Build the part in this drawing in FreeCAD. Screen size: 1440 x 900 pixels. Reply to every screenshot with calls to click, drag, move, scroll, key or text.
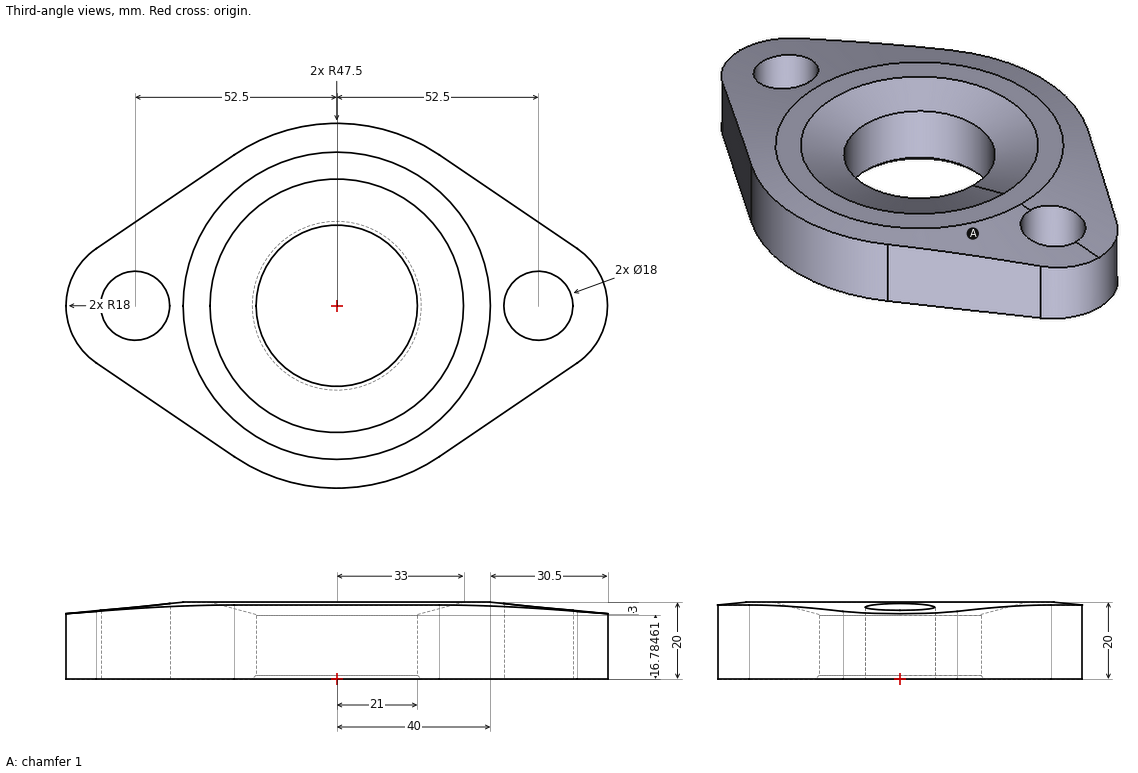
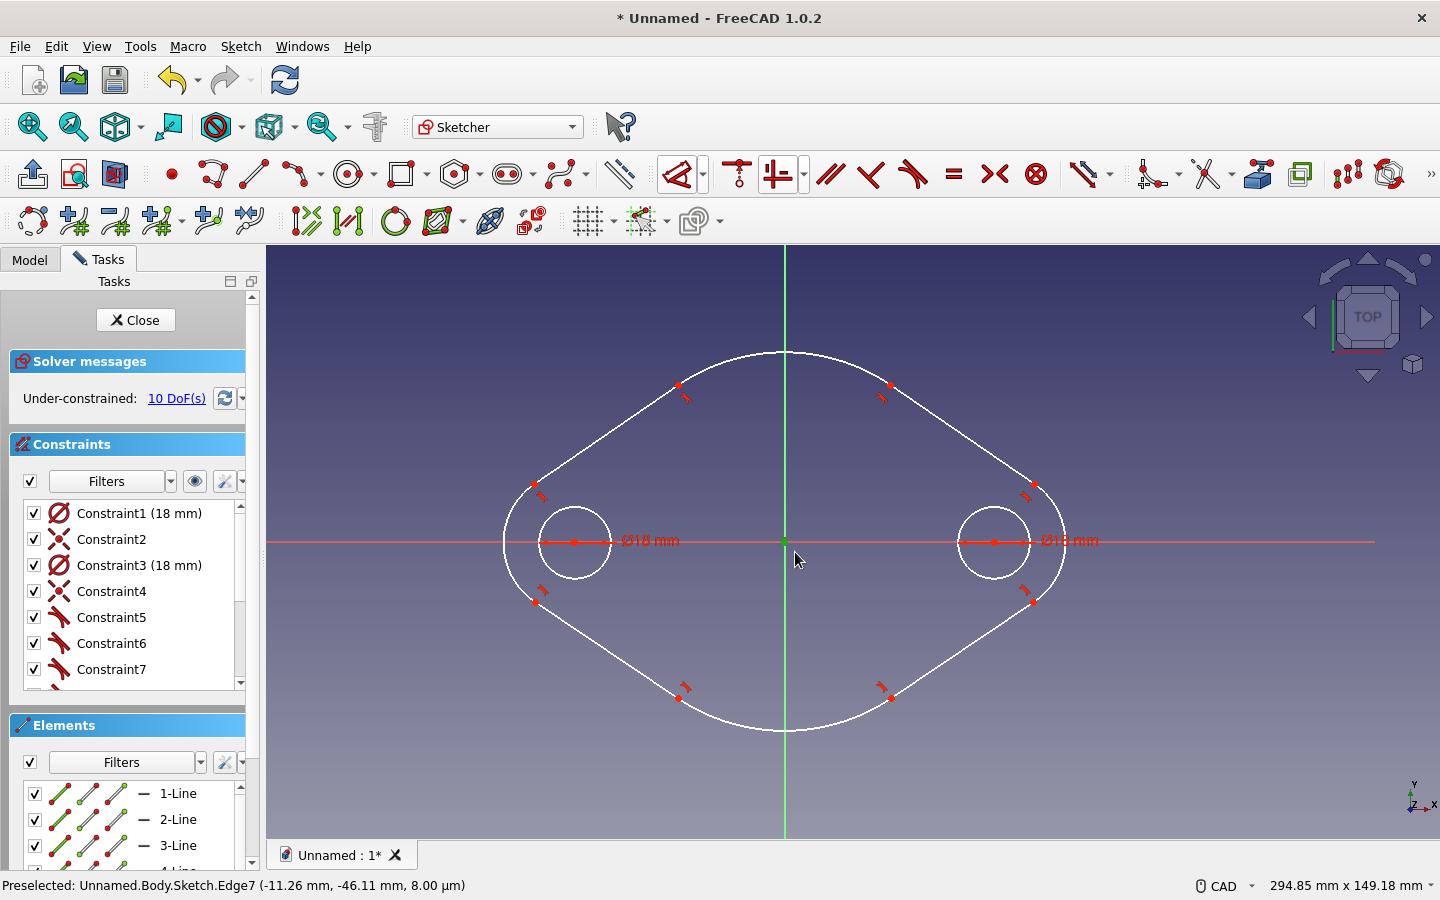
key(c)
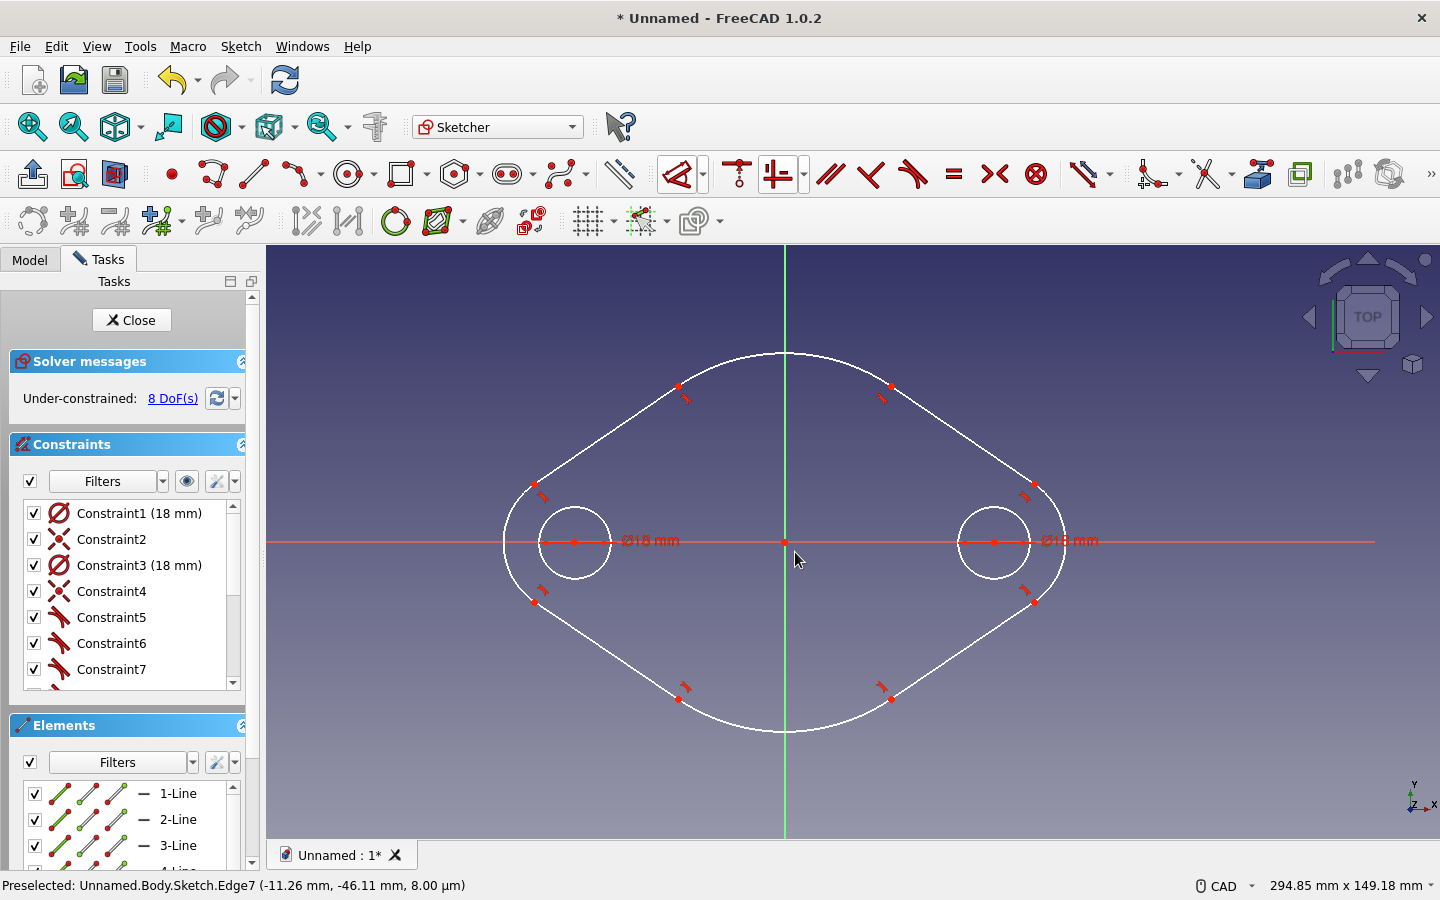
click(829, 359)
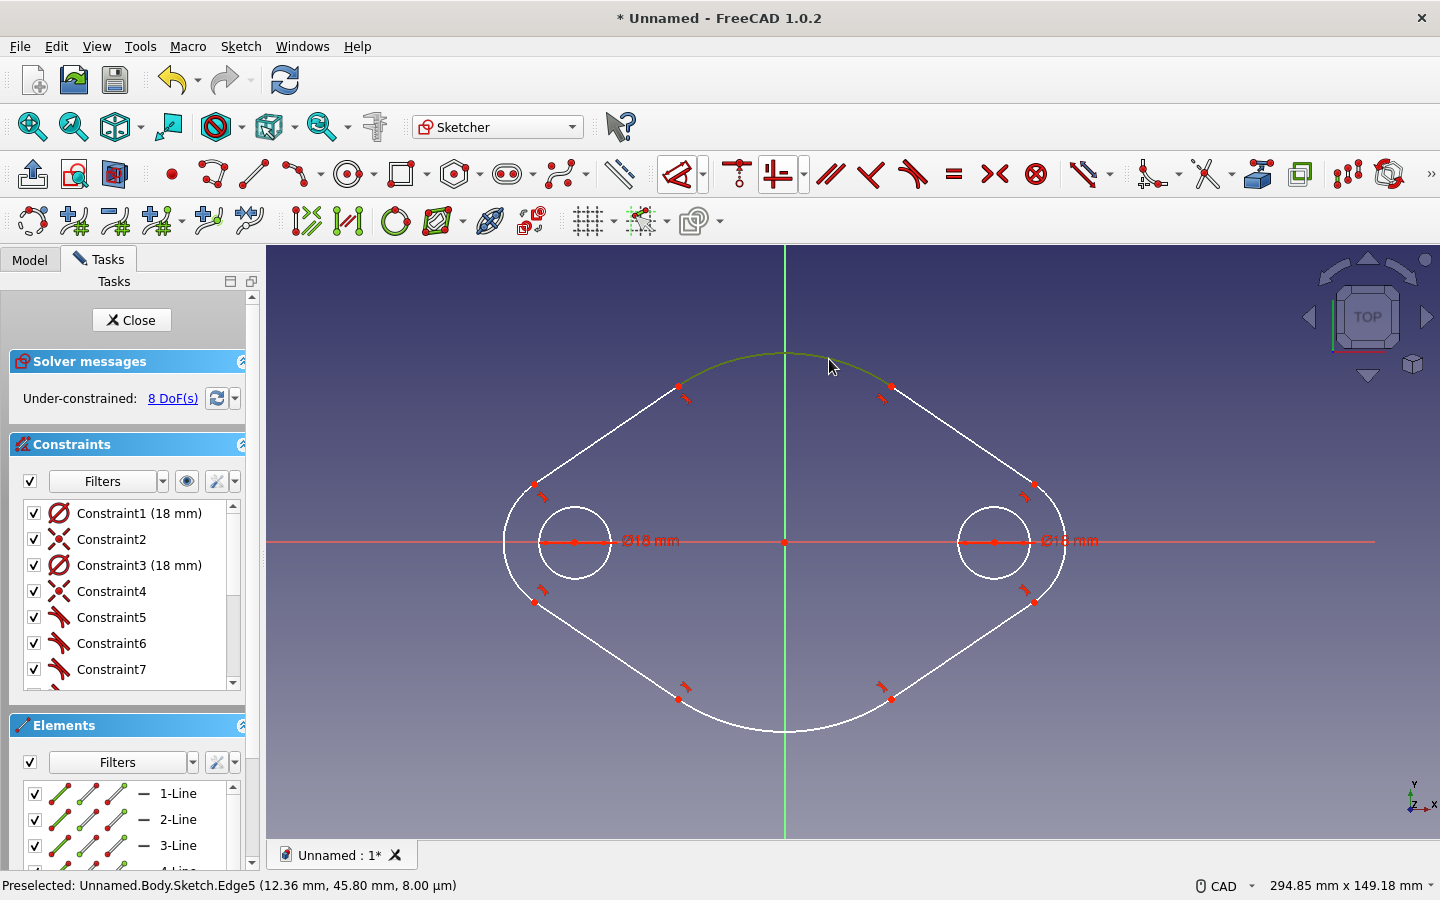
click(740, 726)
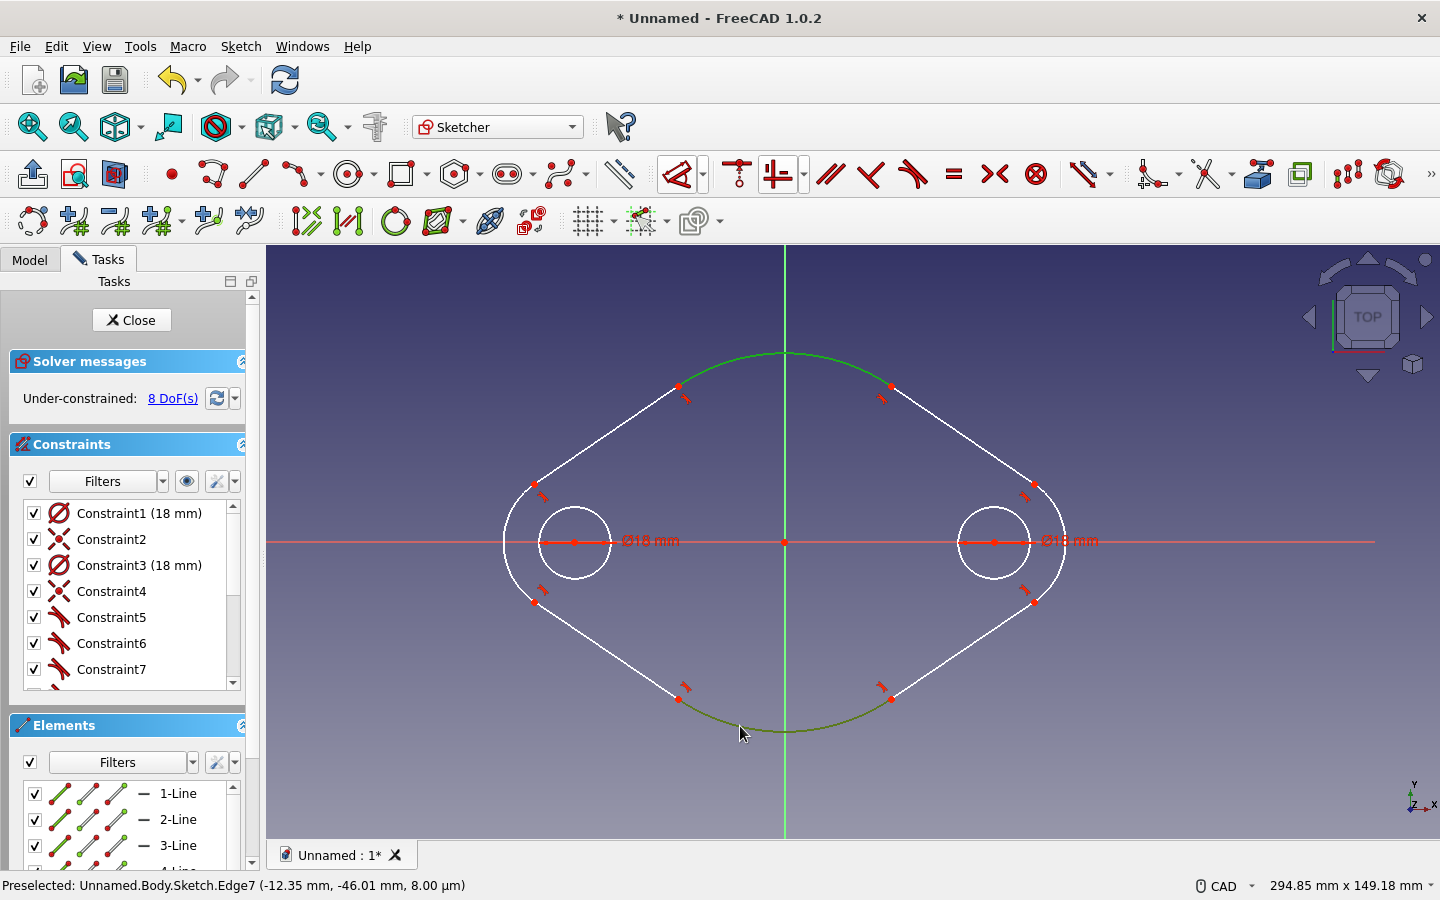
click(954, 174)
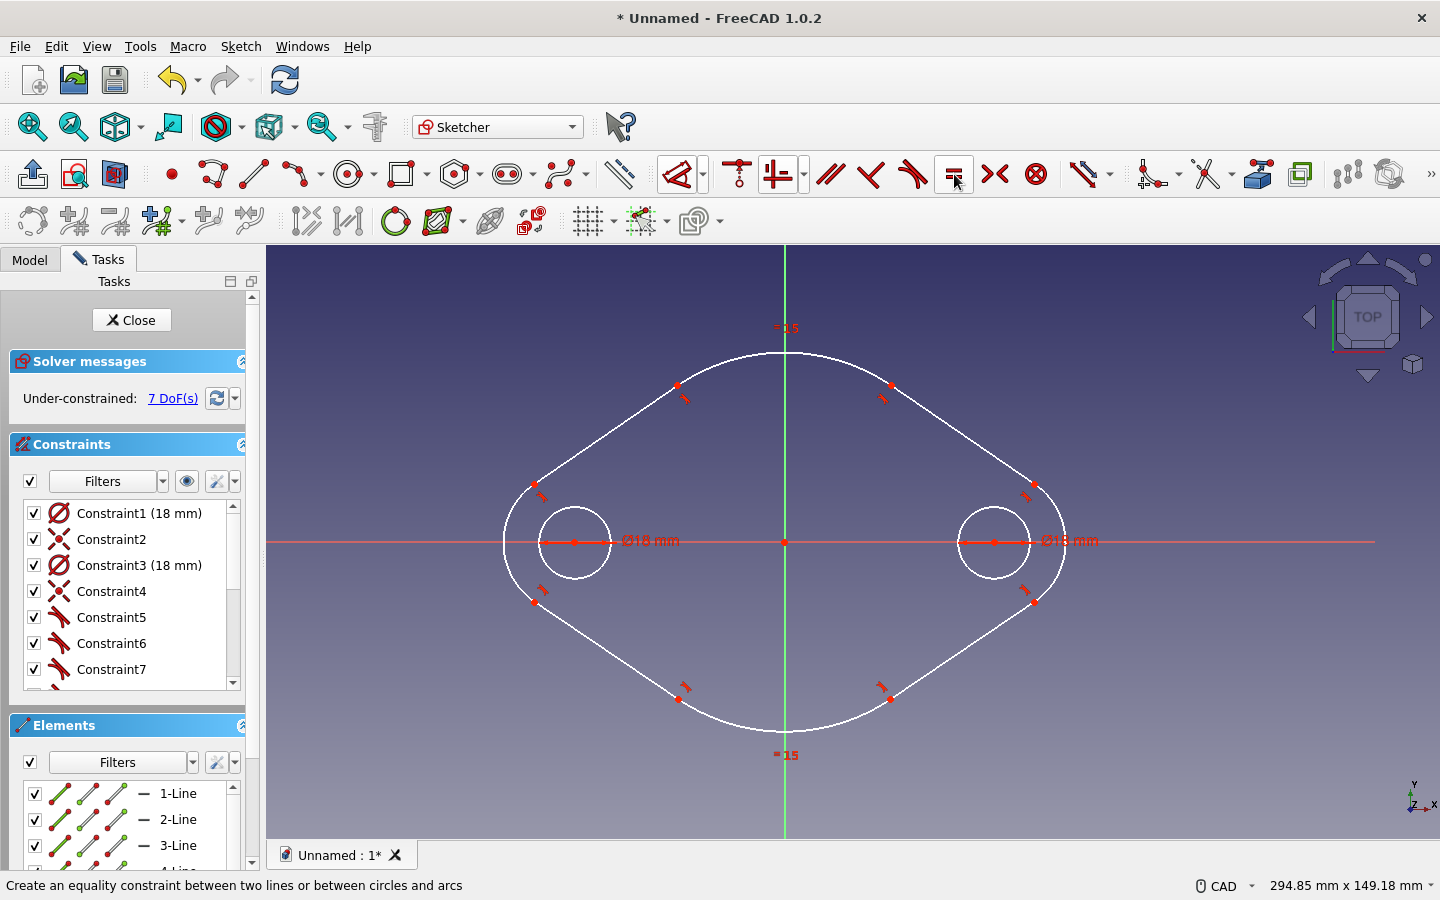
click(509, 516)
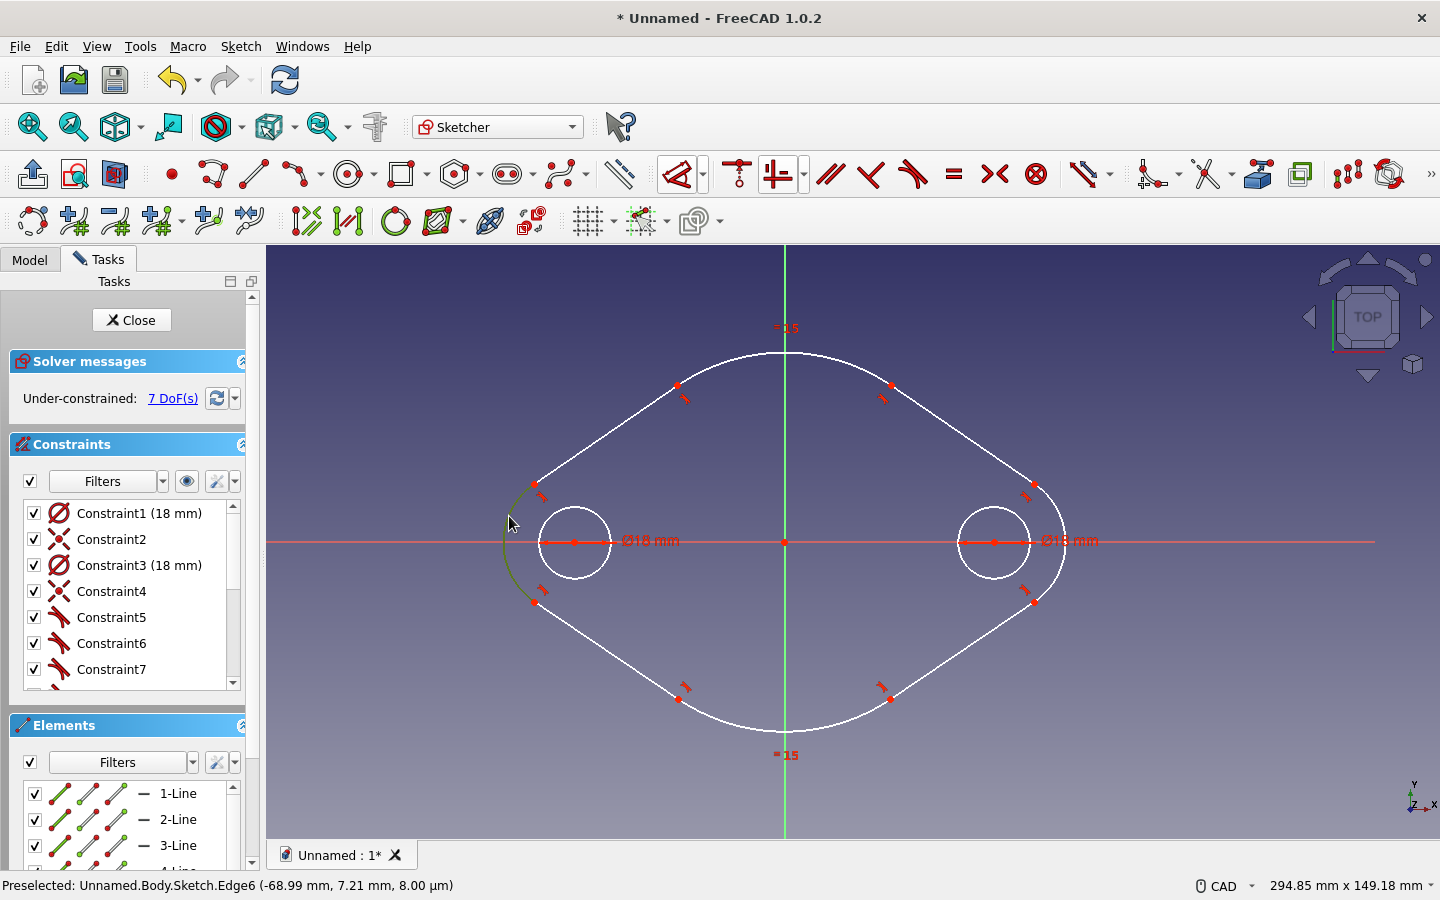
click(1060, 570)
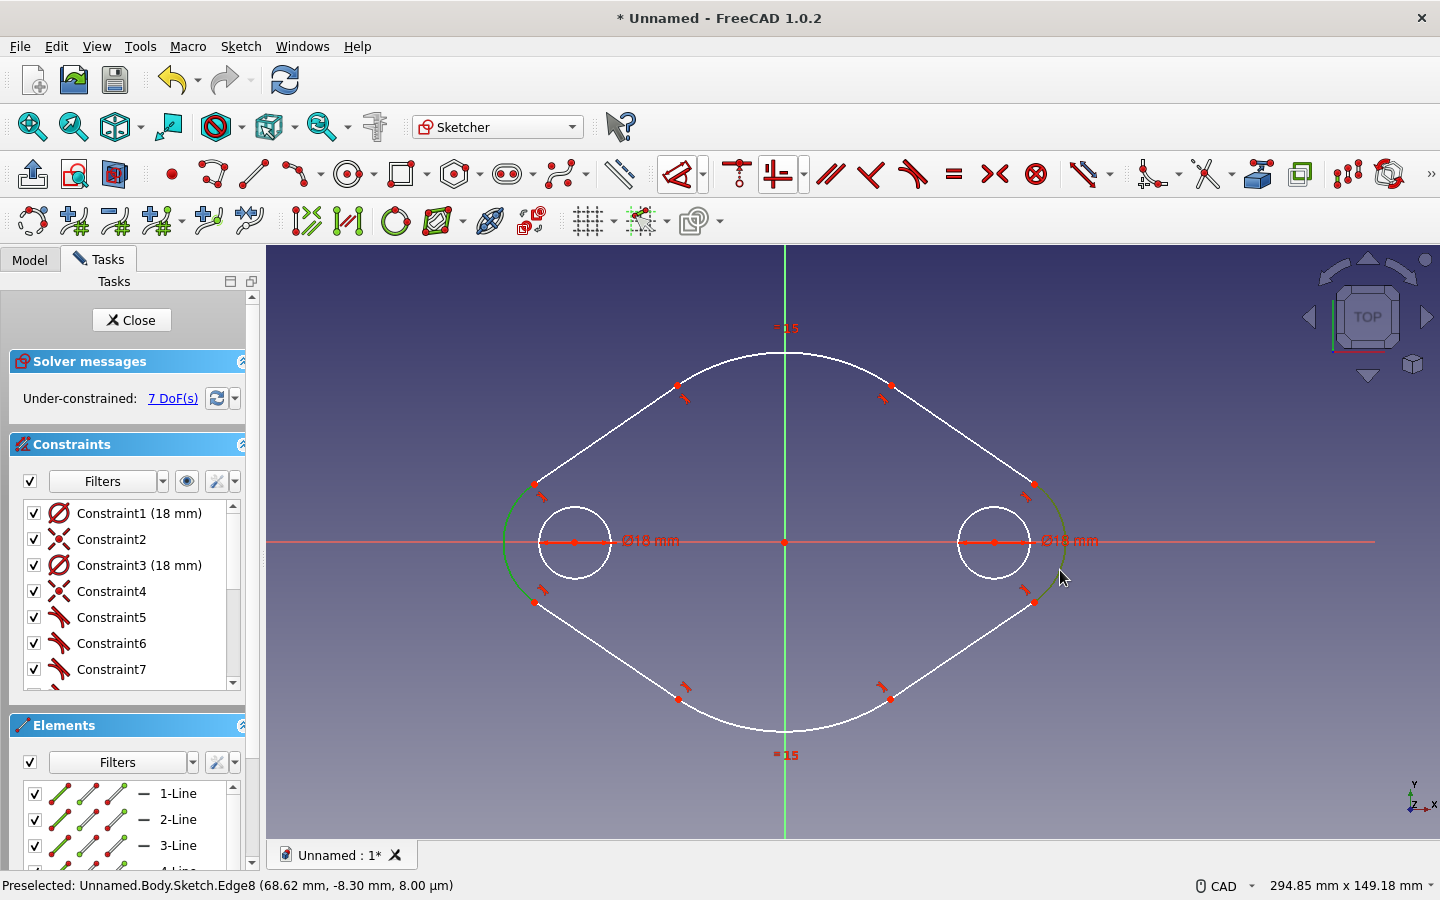
key(e)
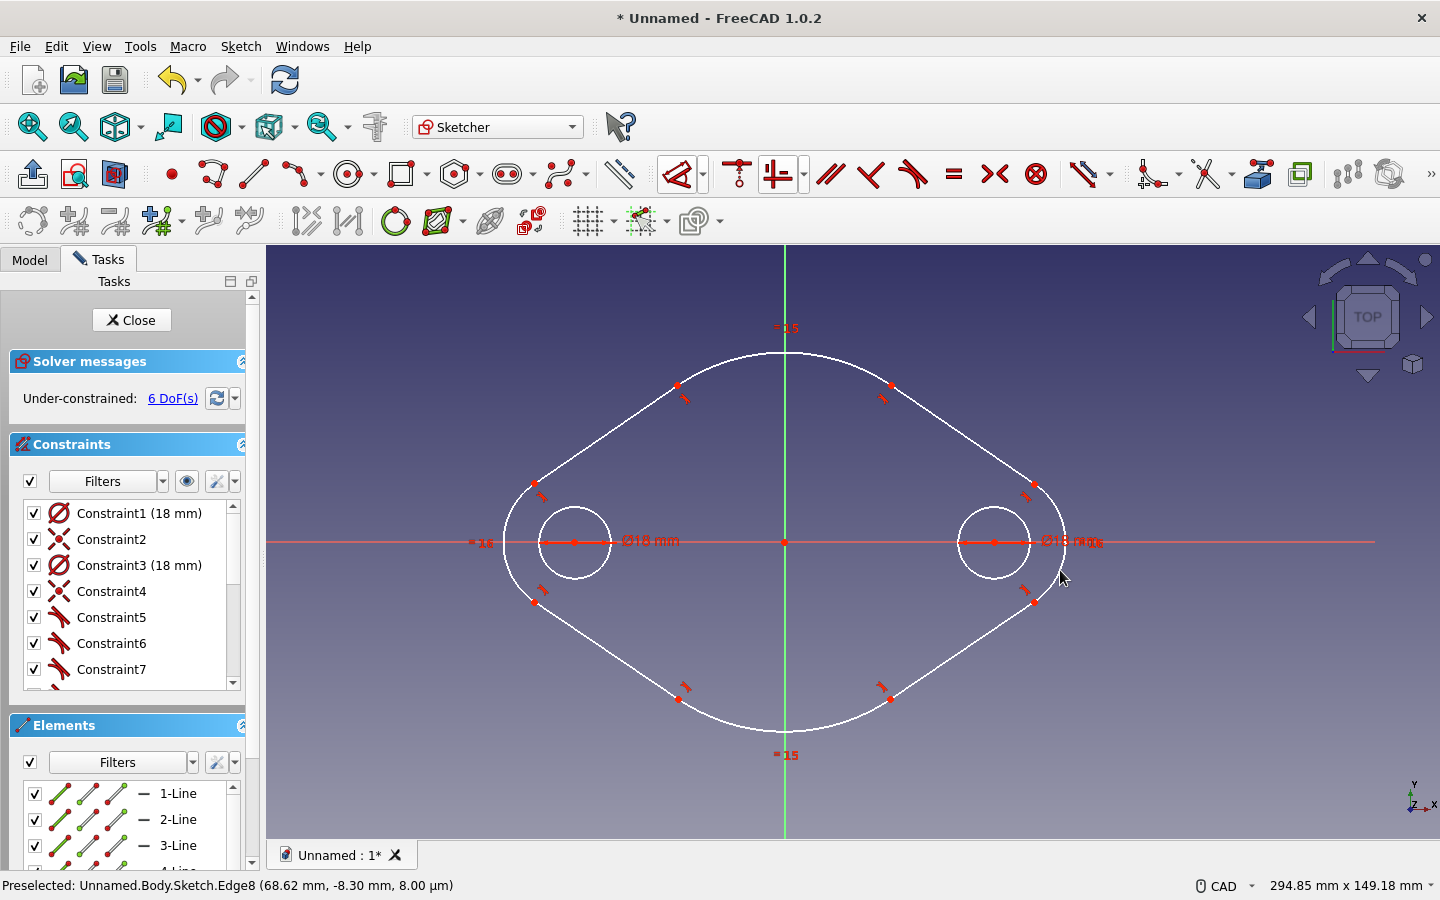
click(575, 543)